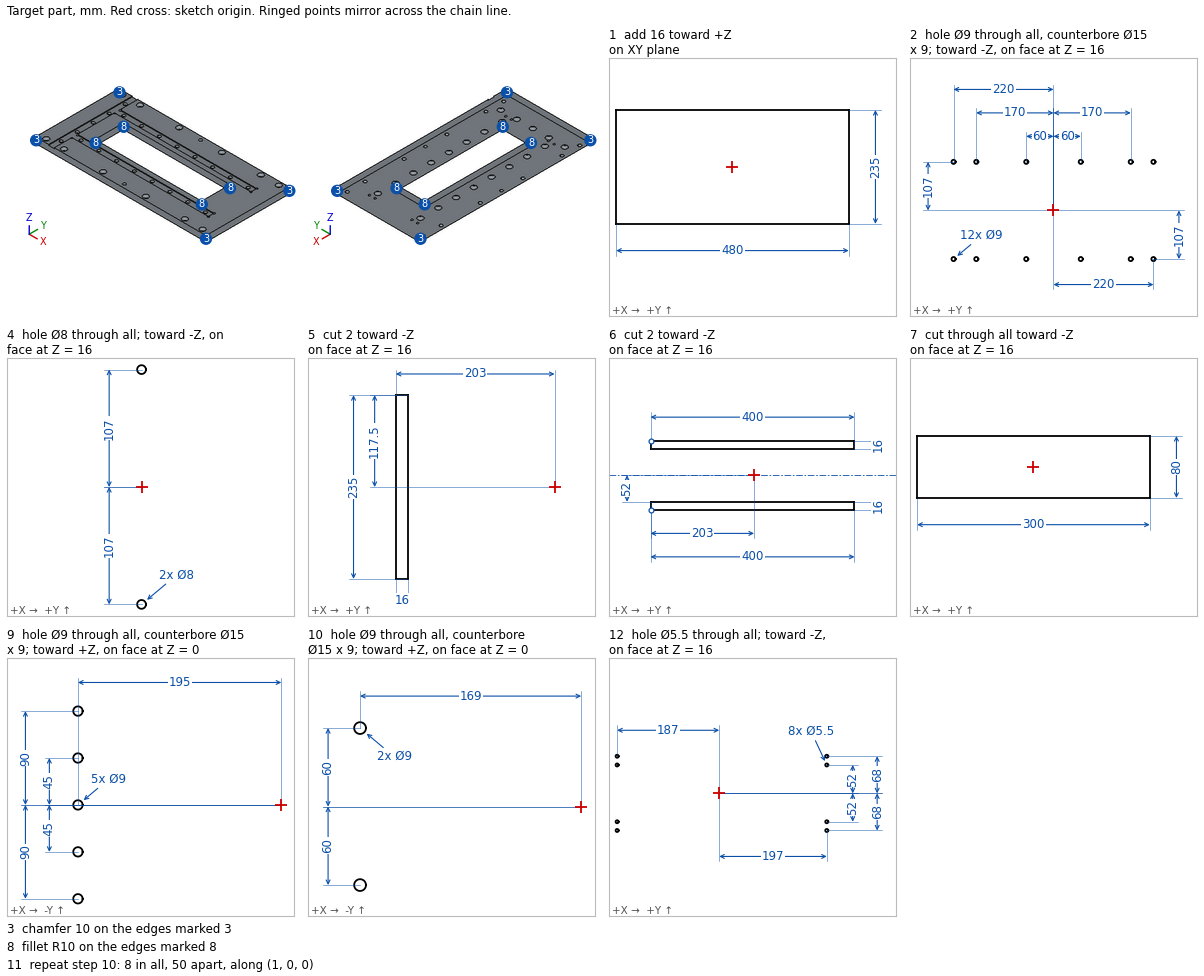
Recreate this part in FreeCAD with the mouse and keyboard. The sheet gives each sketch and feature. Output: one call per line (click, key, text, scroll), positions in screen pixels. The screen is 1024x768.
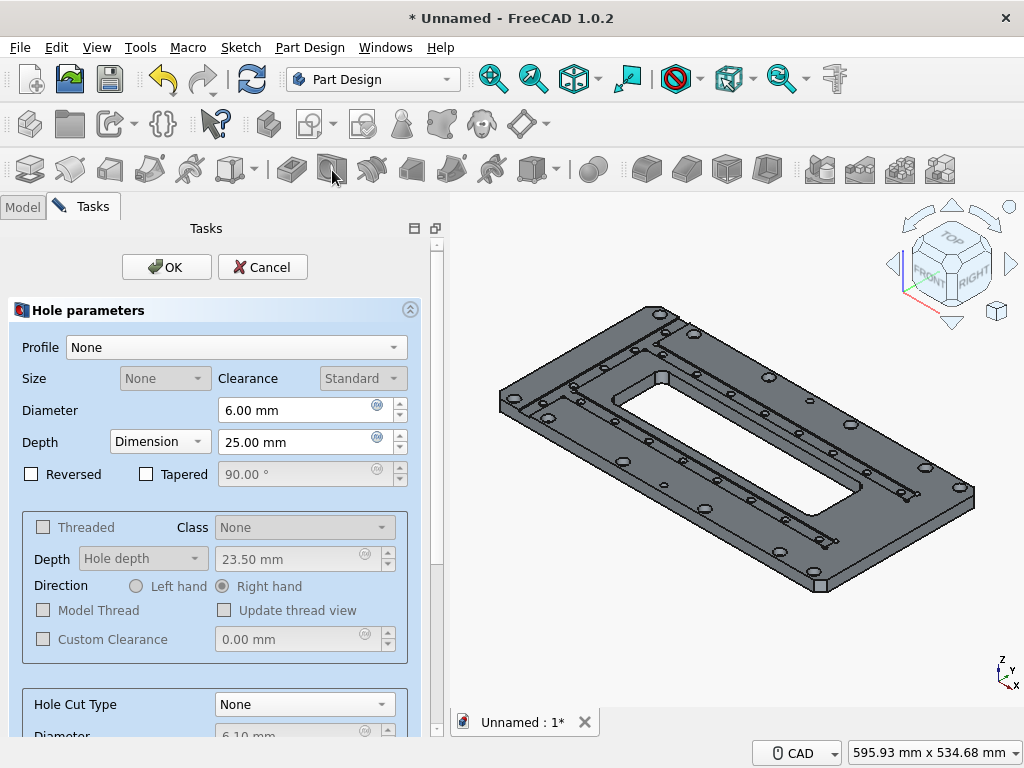
triple_click(305, 410)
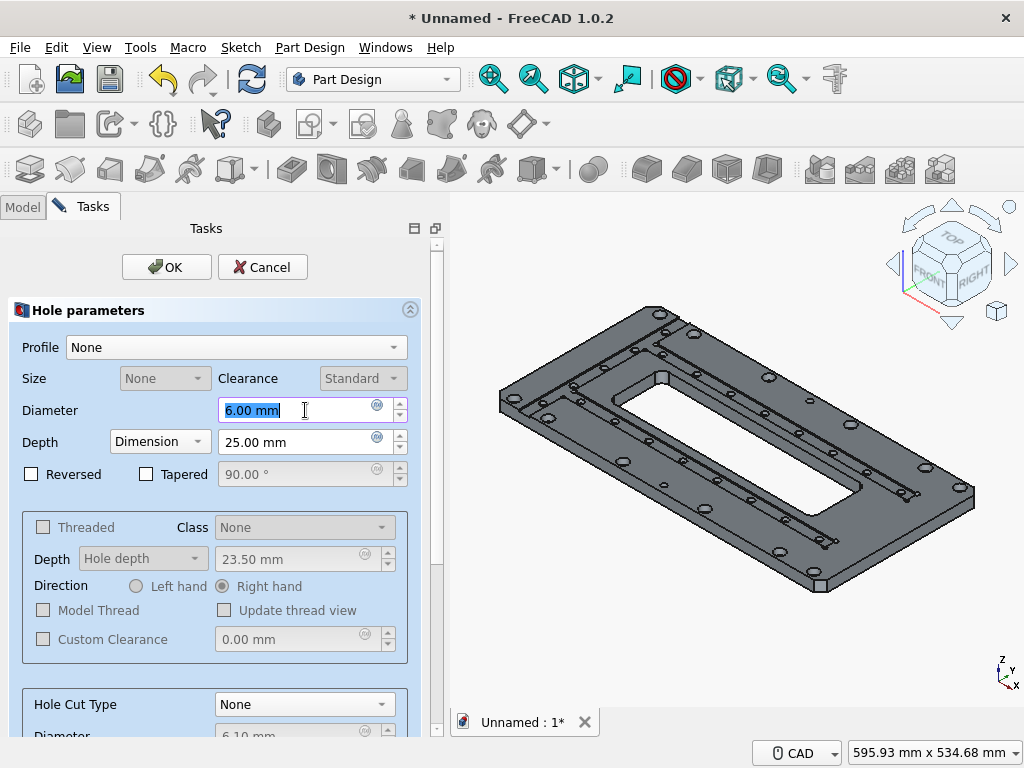
text(5.5)
key(Tab)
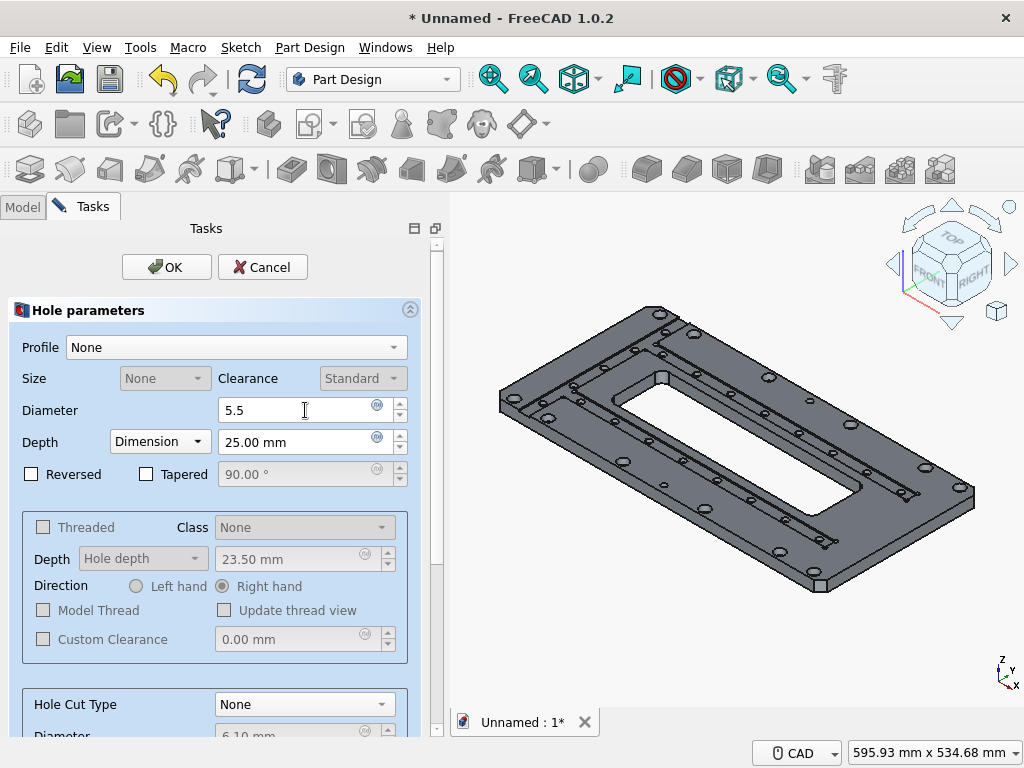
click(161, 442)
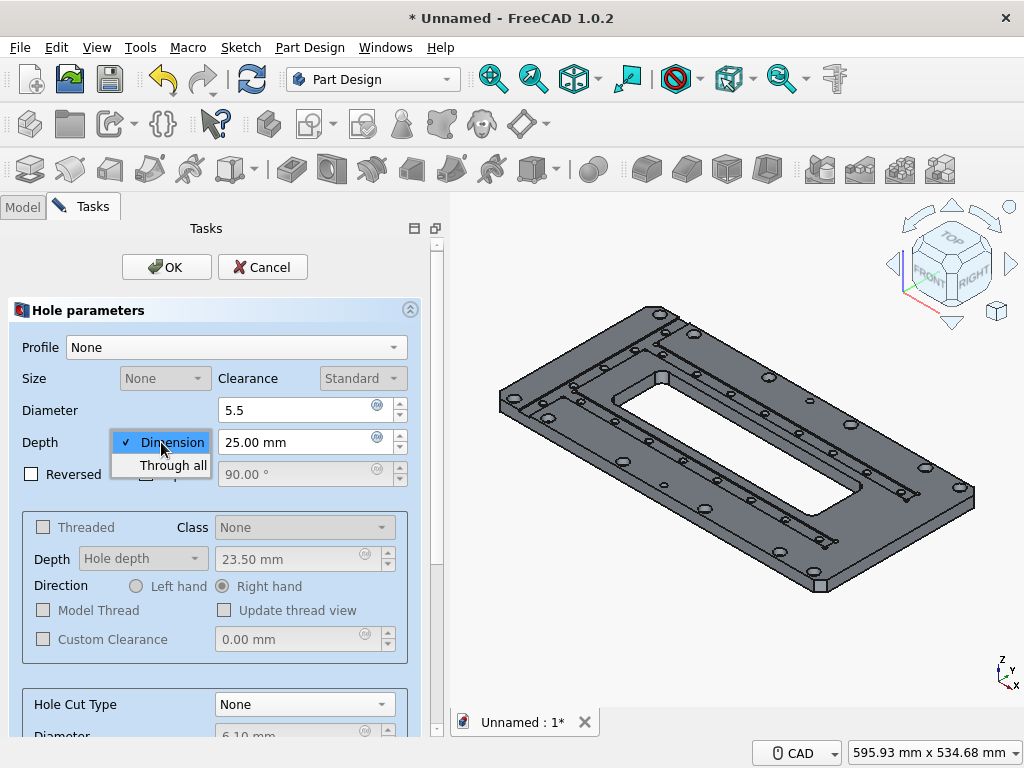
click(160, 466)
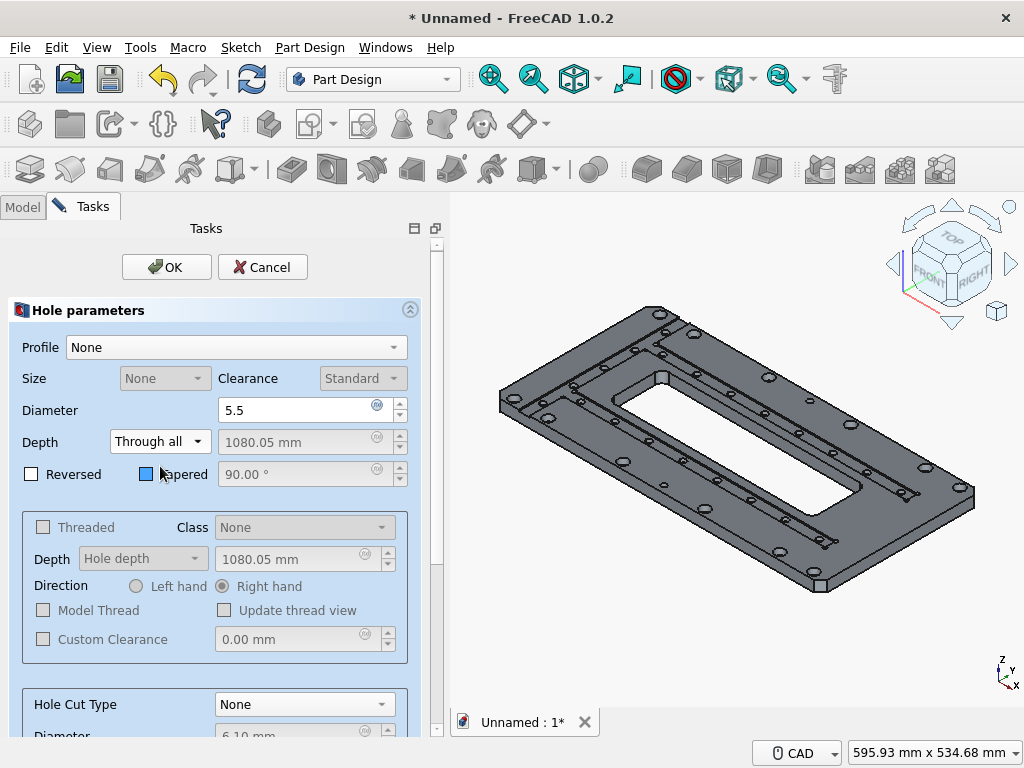
click(167, 267)